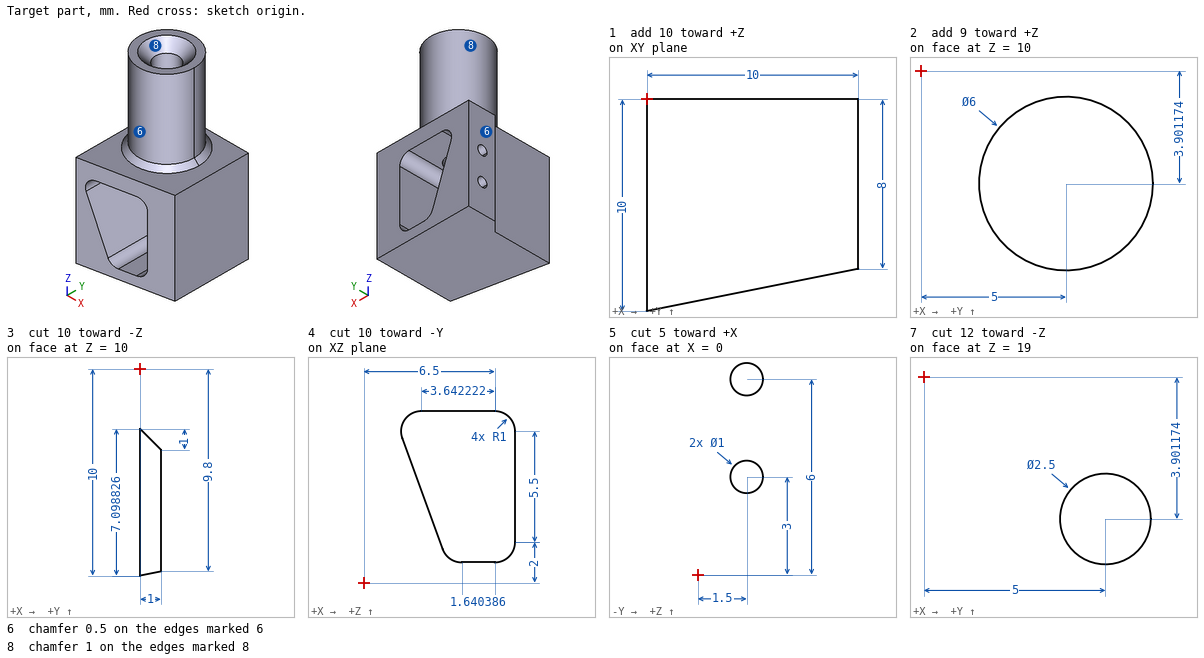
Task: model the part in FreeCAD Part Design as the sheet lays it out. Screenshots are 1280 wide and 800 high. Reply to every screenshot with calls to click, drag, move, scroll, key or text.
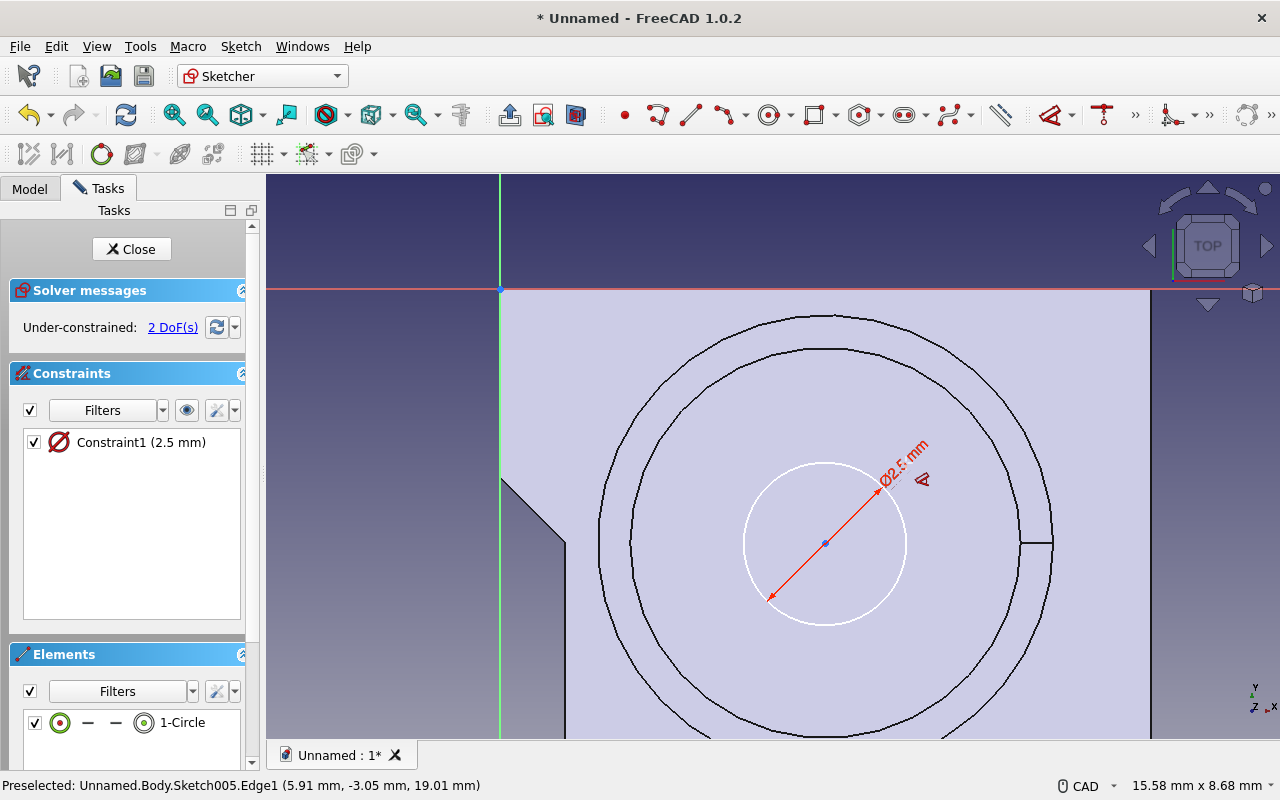
click(825, 544)
click(663, 255)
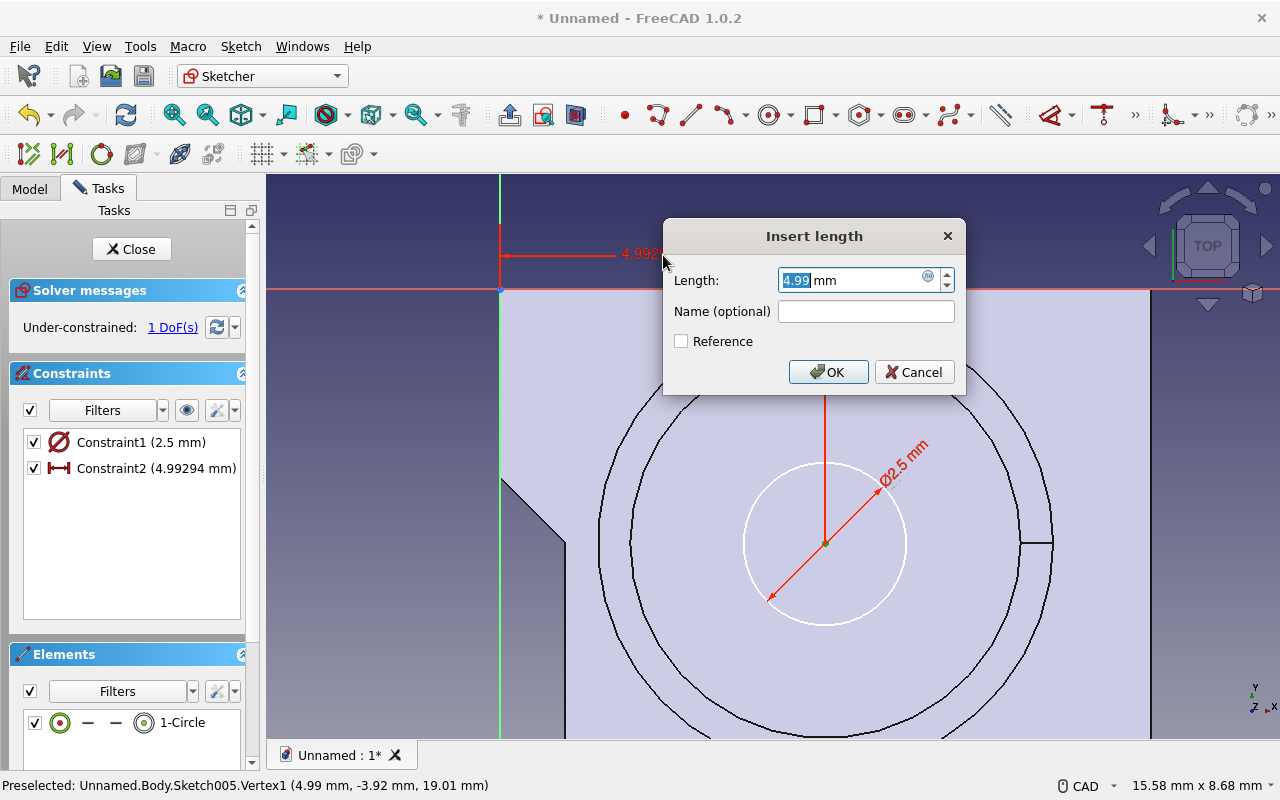
text(5)
key(Return)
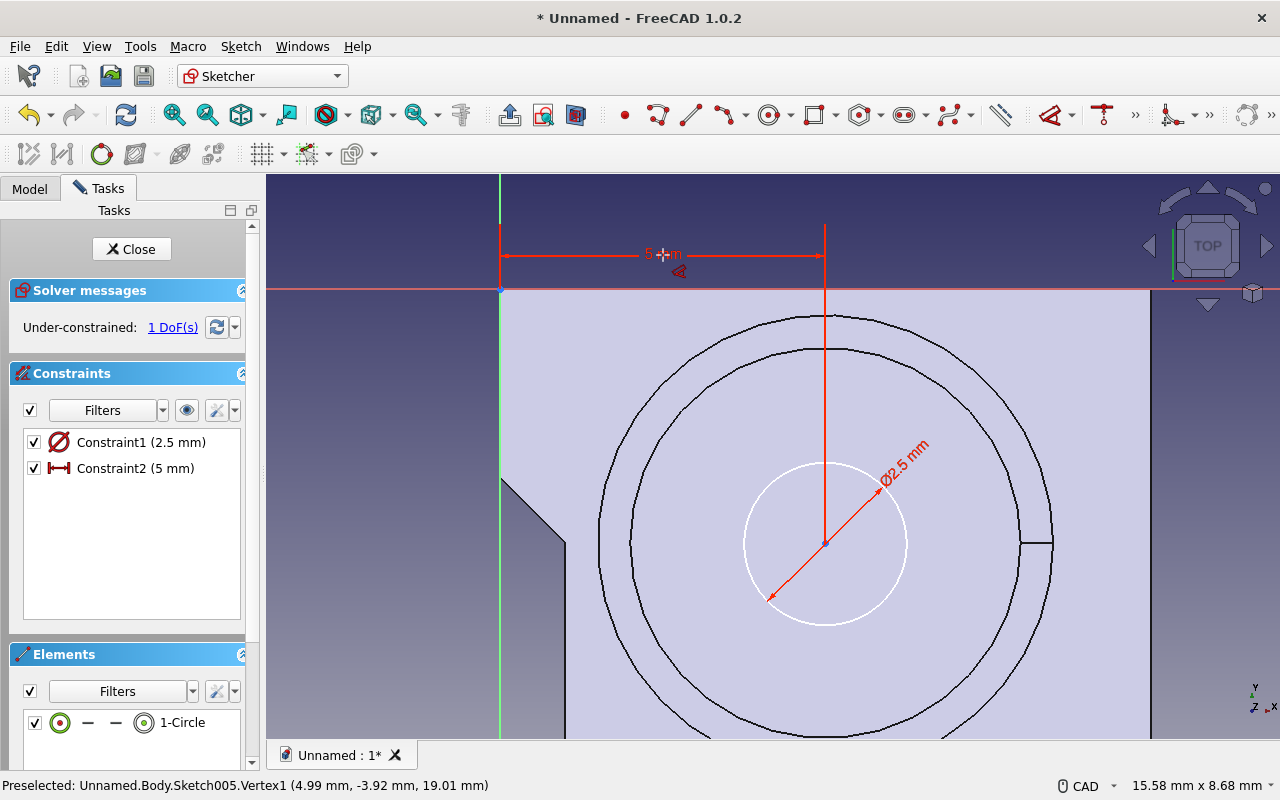
click(825, 544)
click(466, 417)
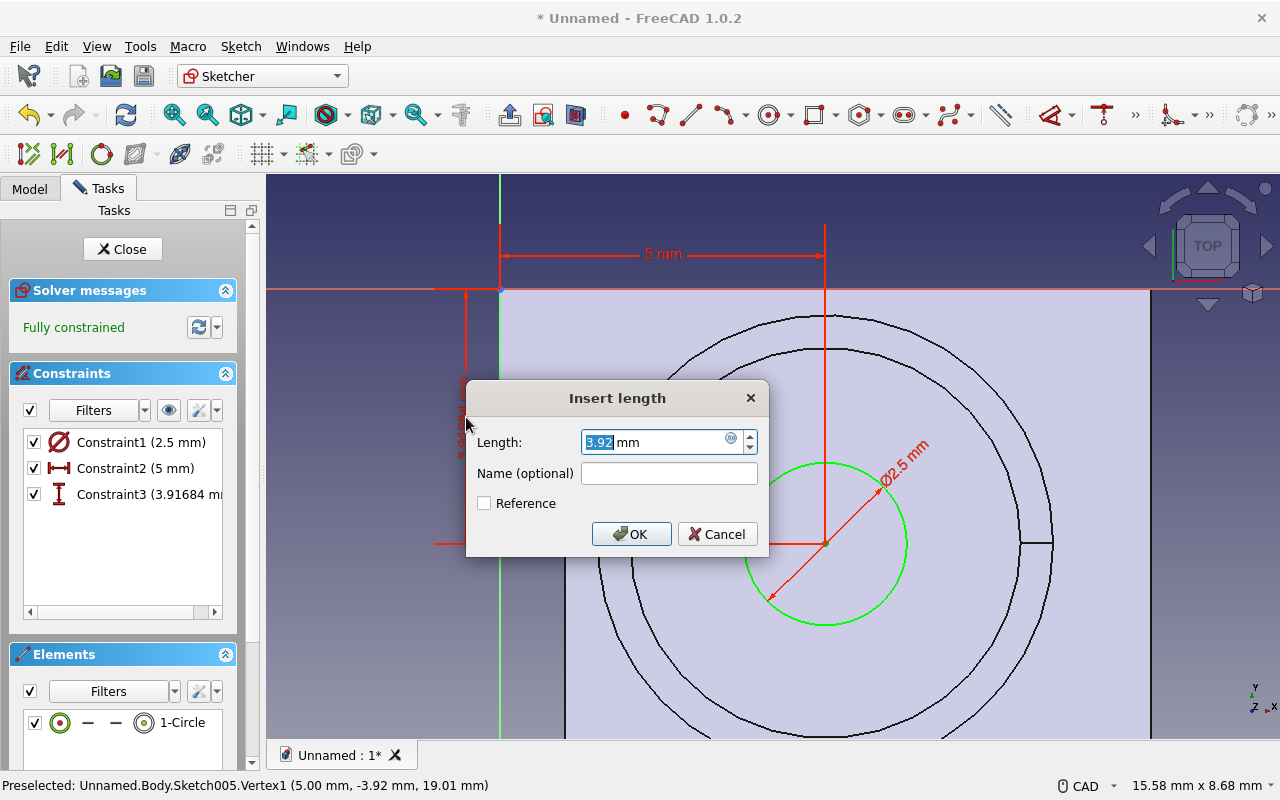
text(3.901174)
key(Return)
key(Escape)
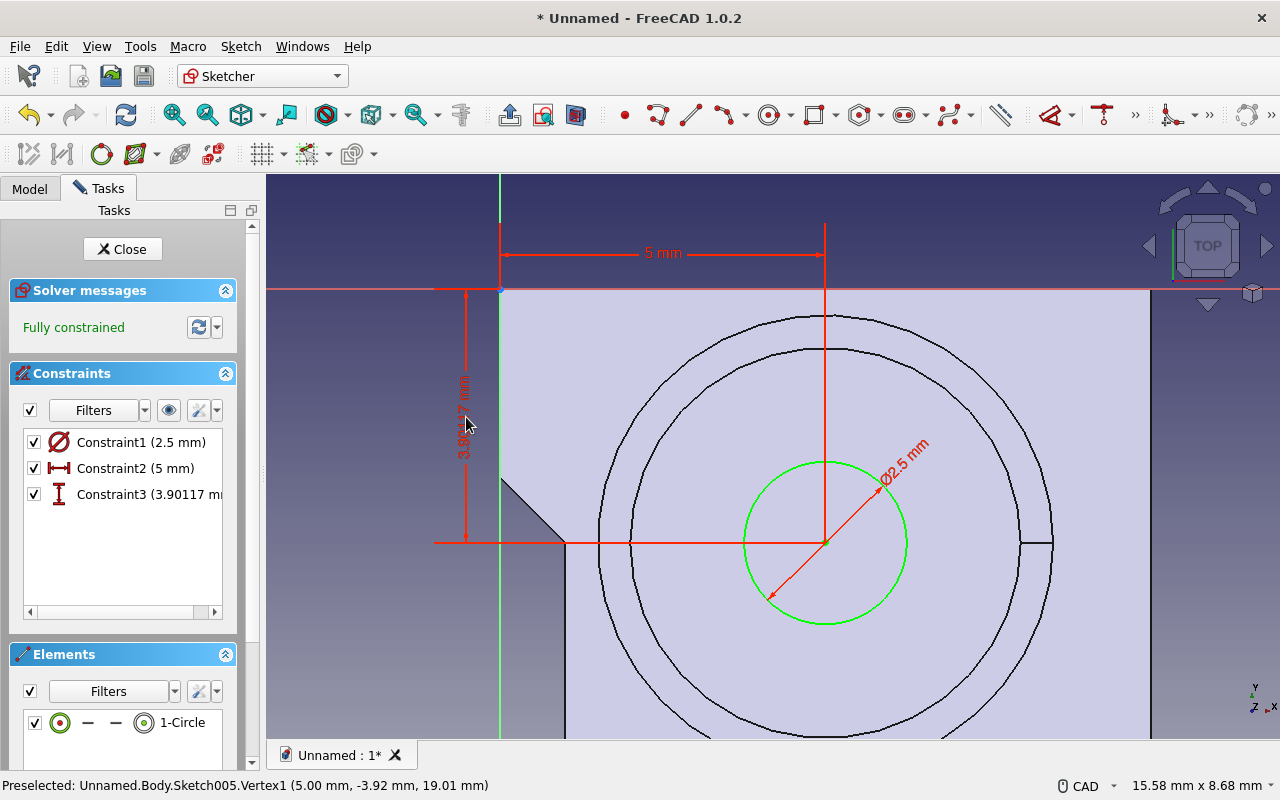
click(123, 249)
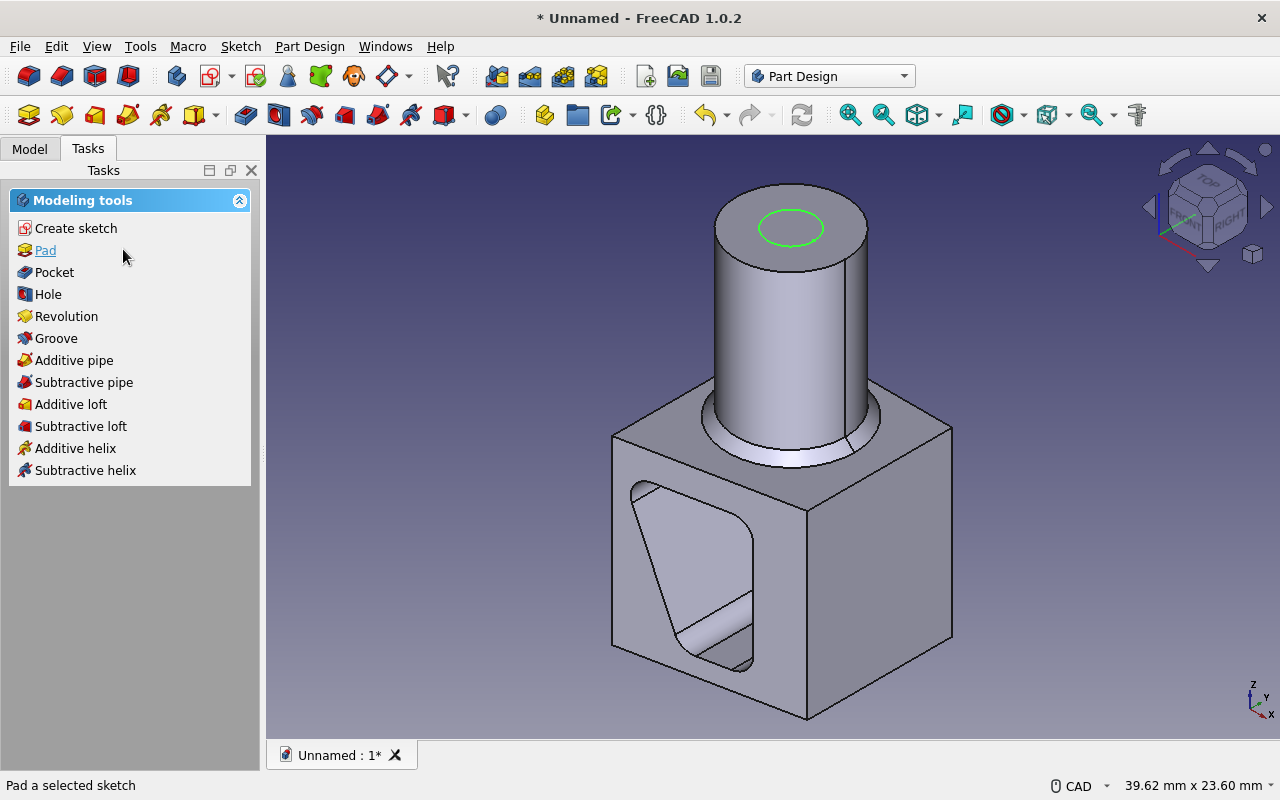
click(246, 116)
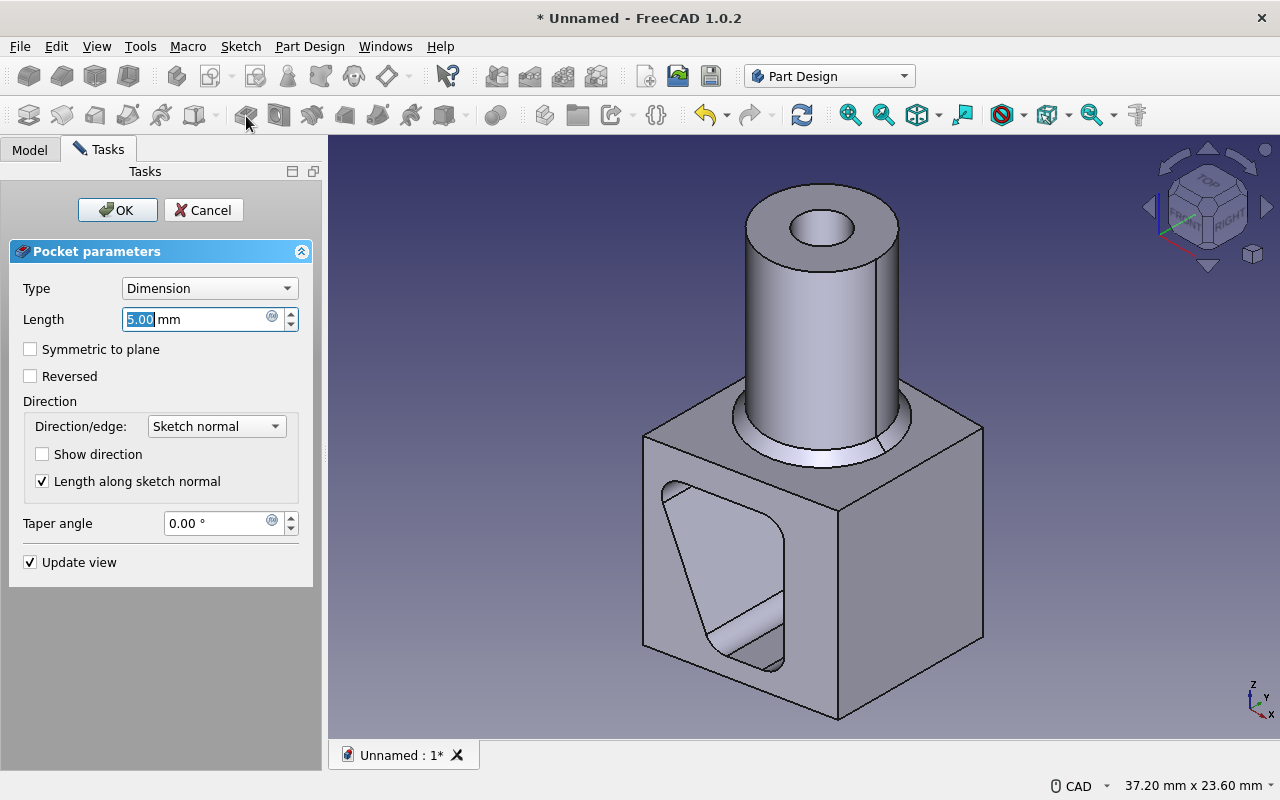
text(12)
key(Tab)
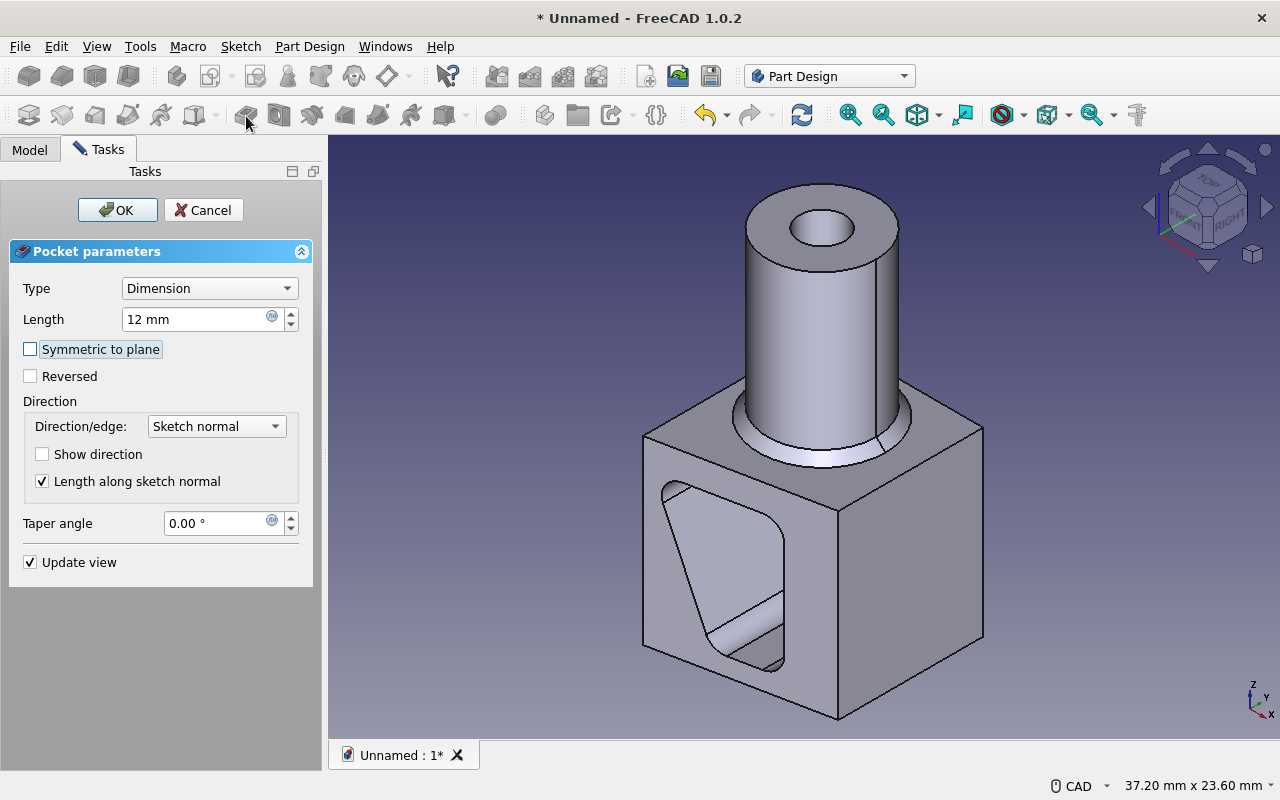
click(118, 210)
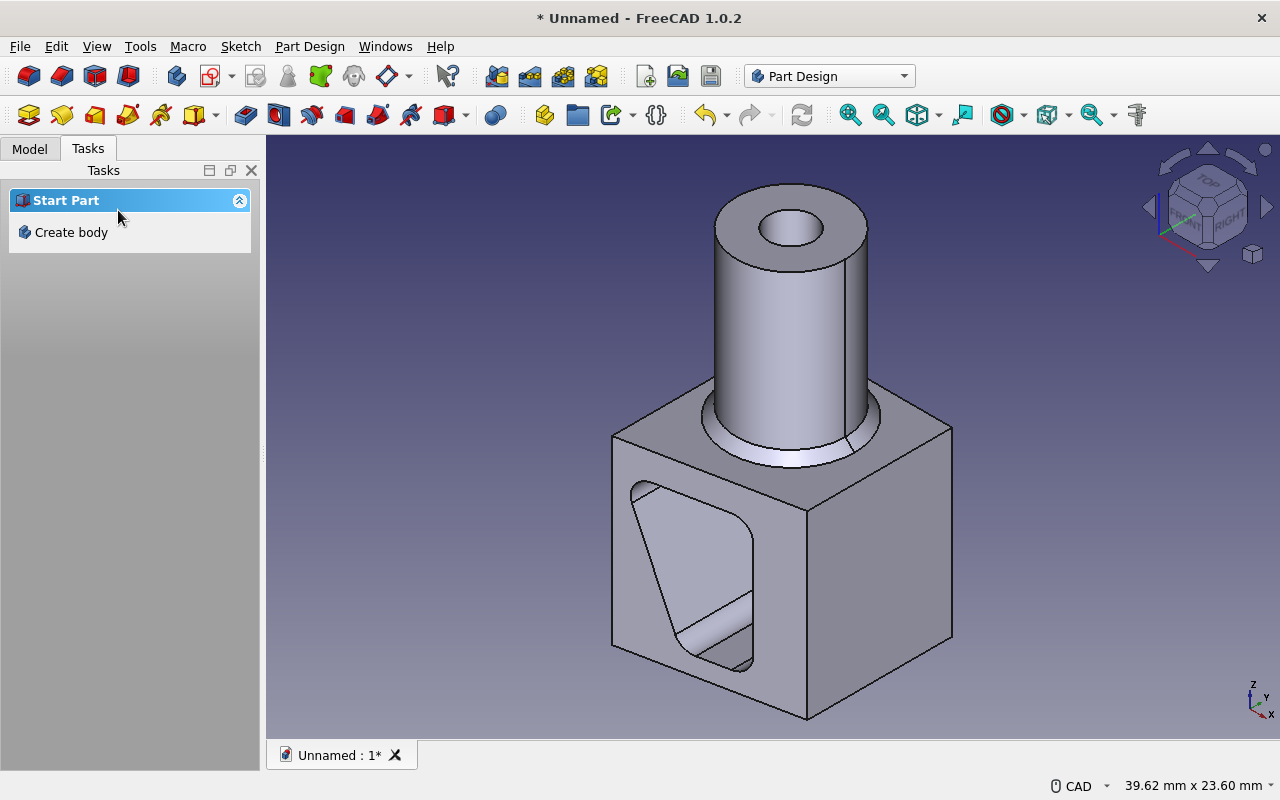
key(v)
key(f)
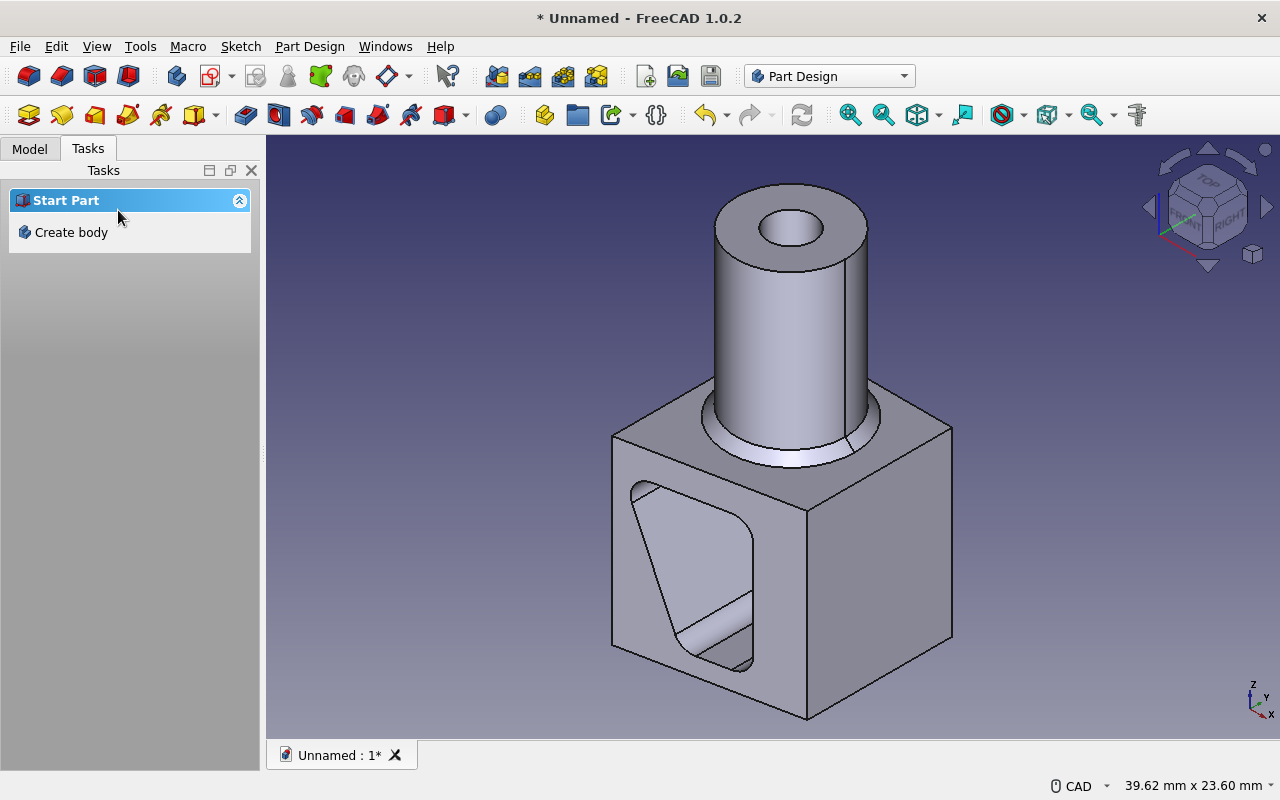
click(768, 214)